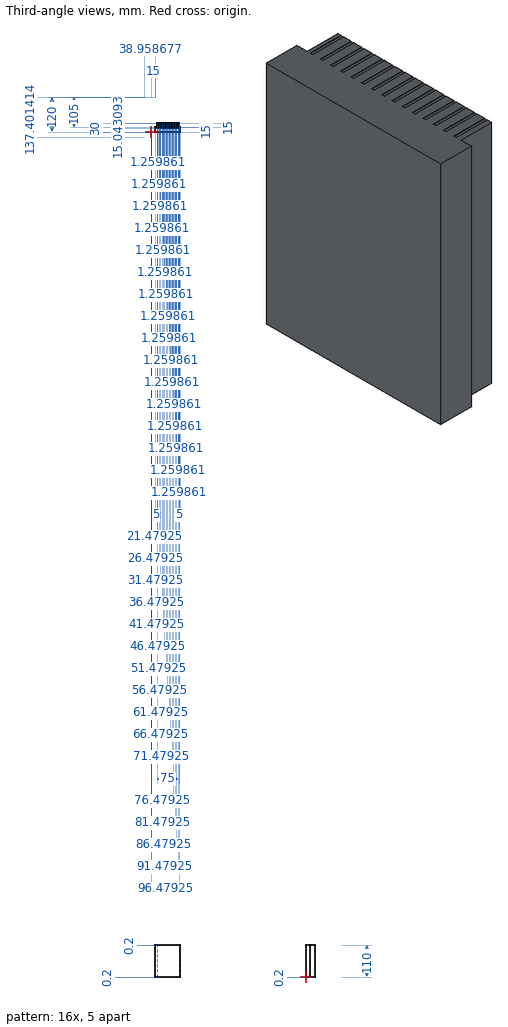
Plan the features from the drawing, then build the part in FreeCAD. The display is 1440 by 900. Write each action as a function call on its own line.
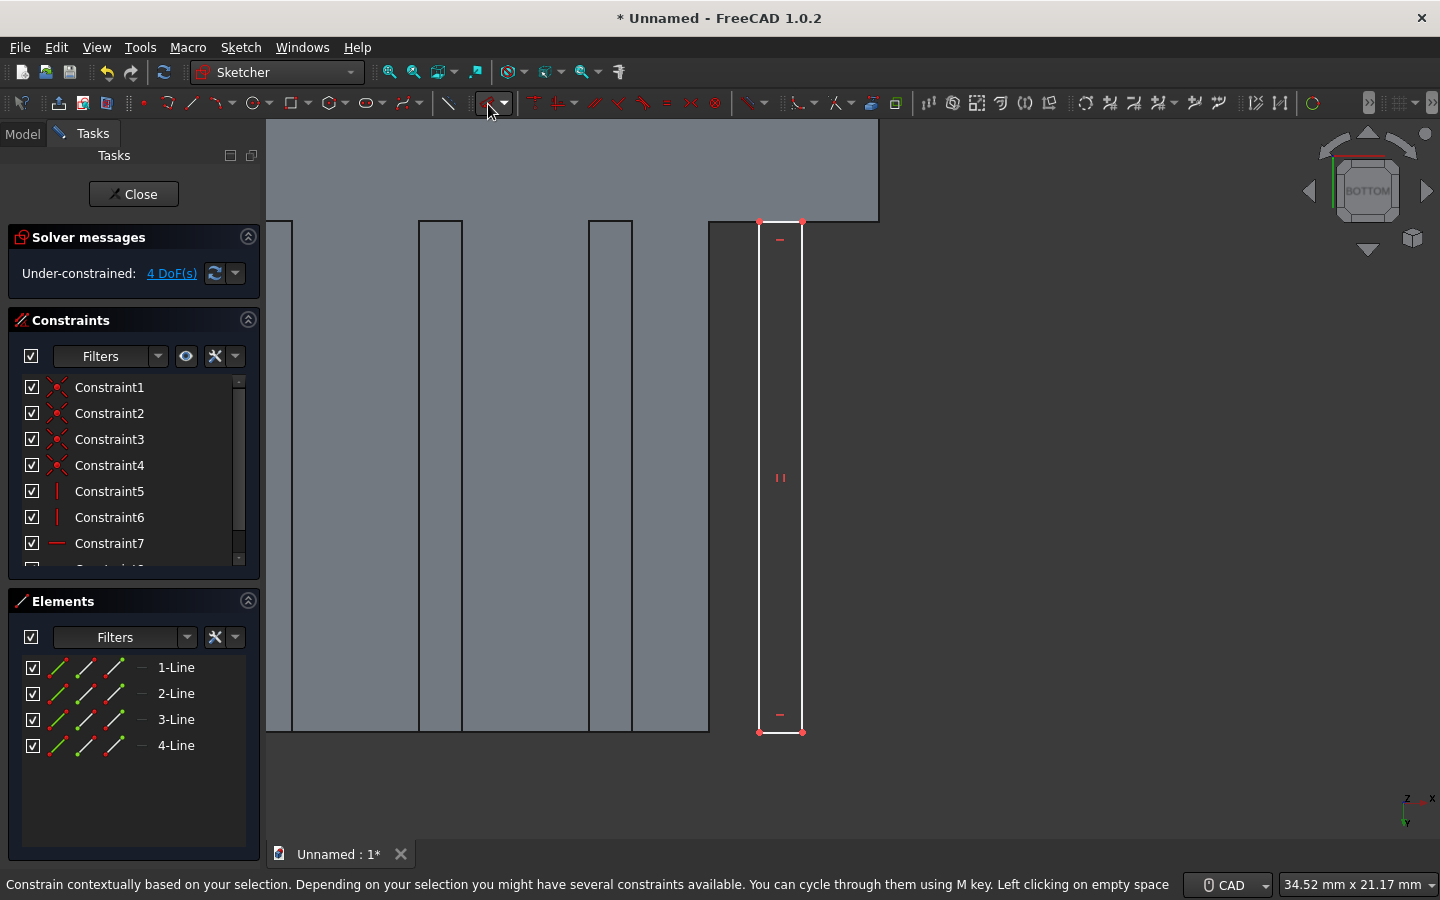
click(759, 733)
click(817, 440)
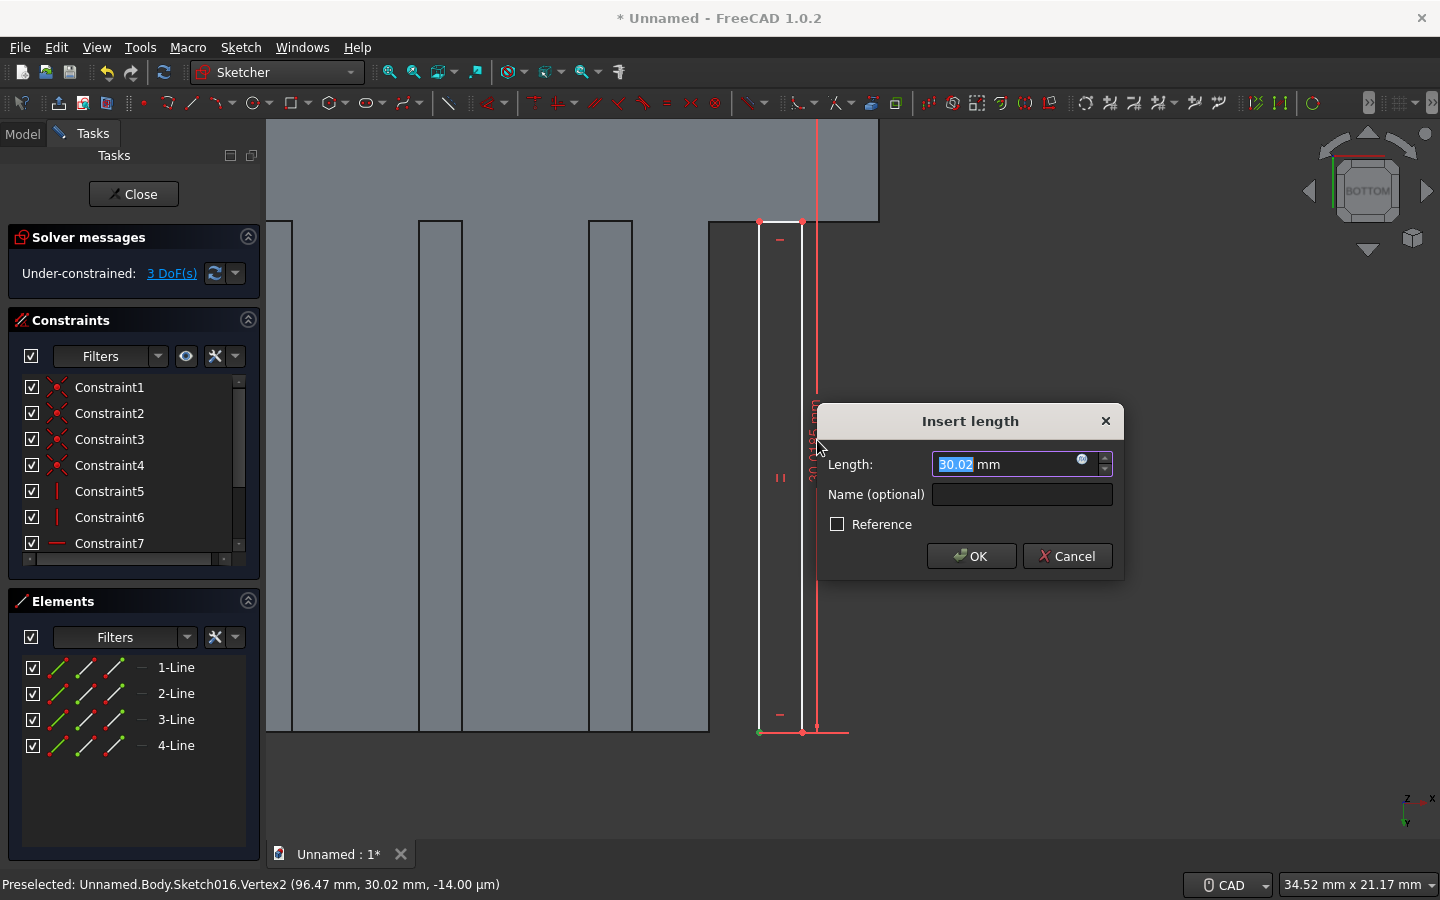
text(30)
key(Return)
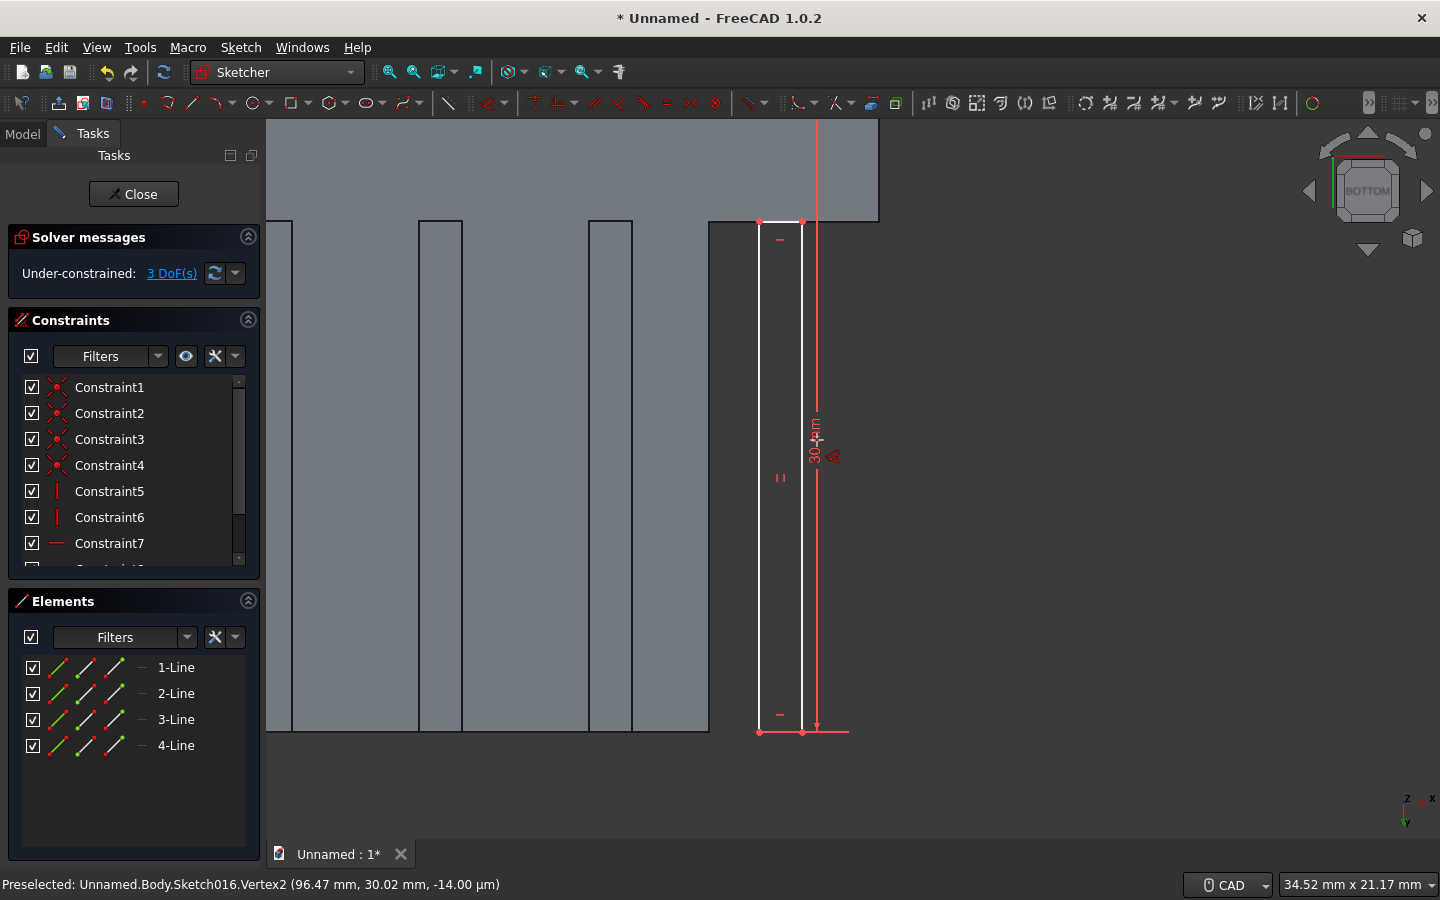
click(772, 732)
click(781, 766)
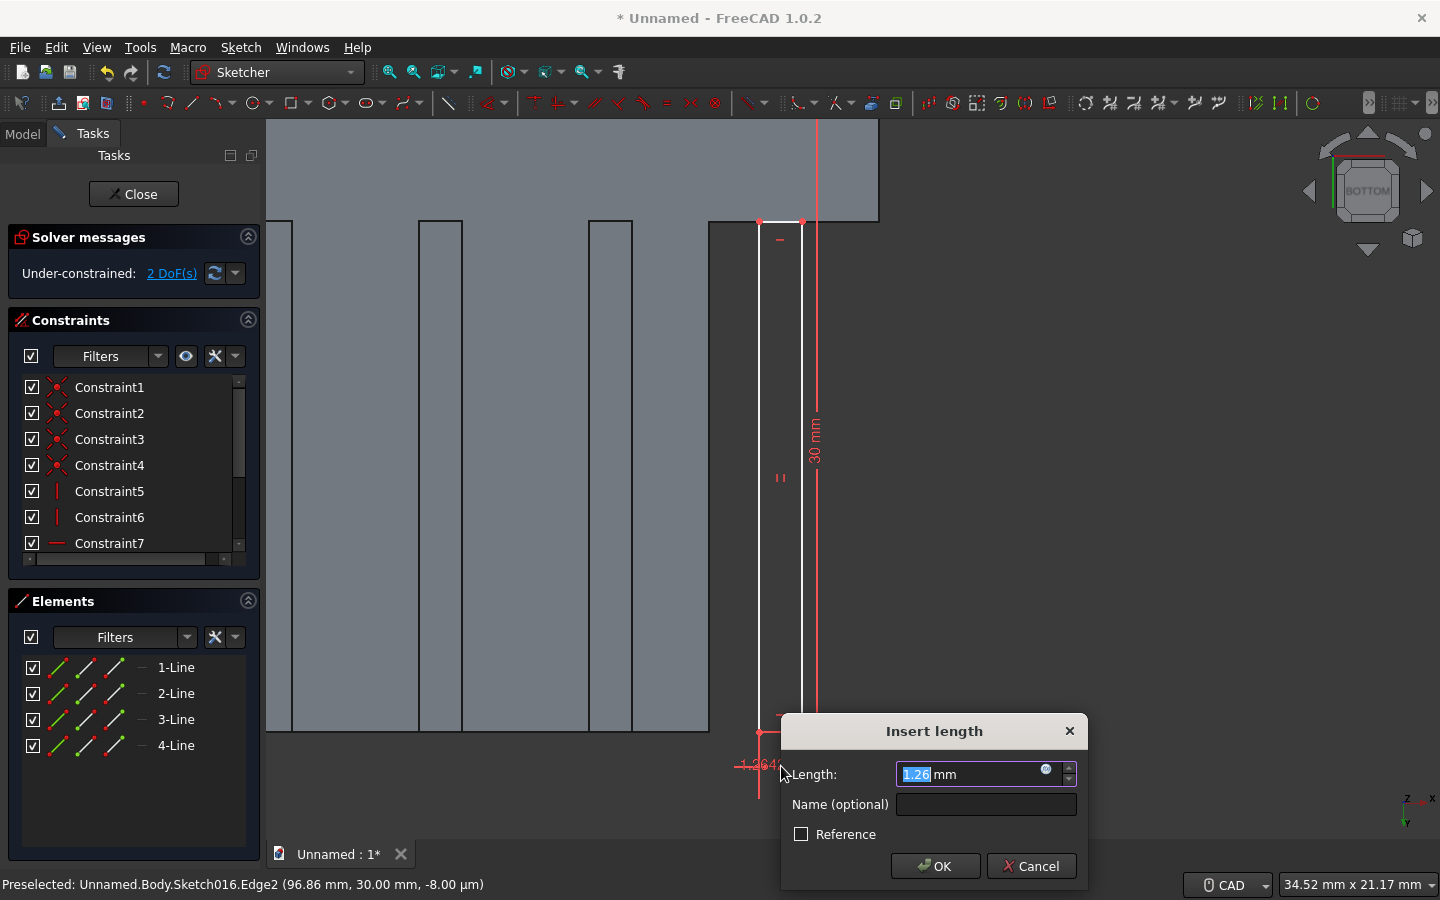
text(1.259861)
key(Return)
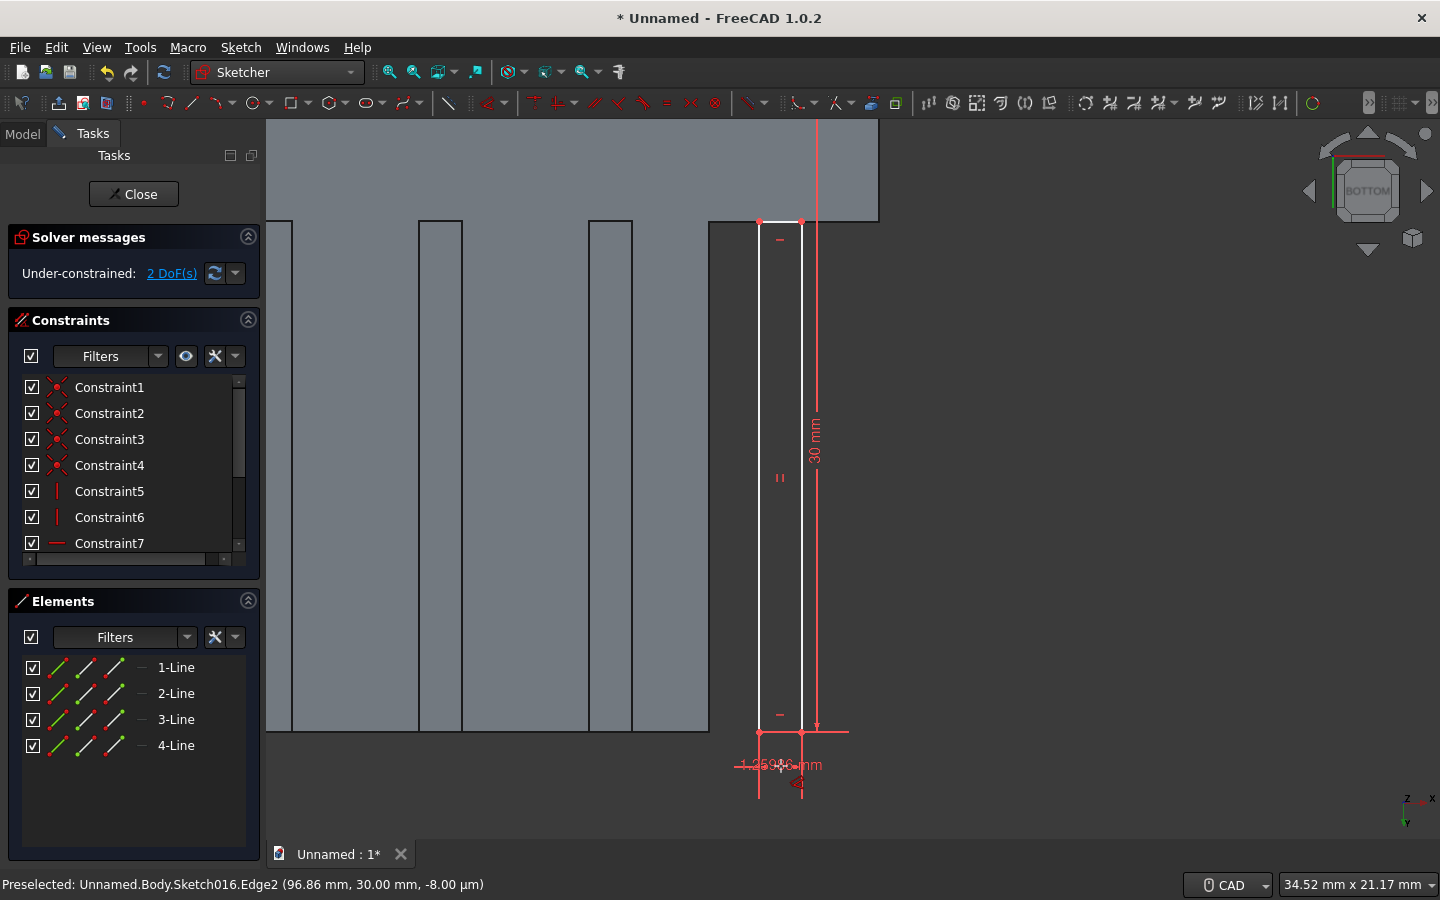
click(759, 375)
click(725, 477)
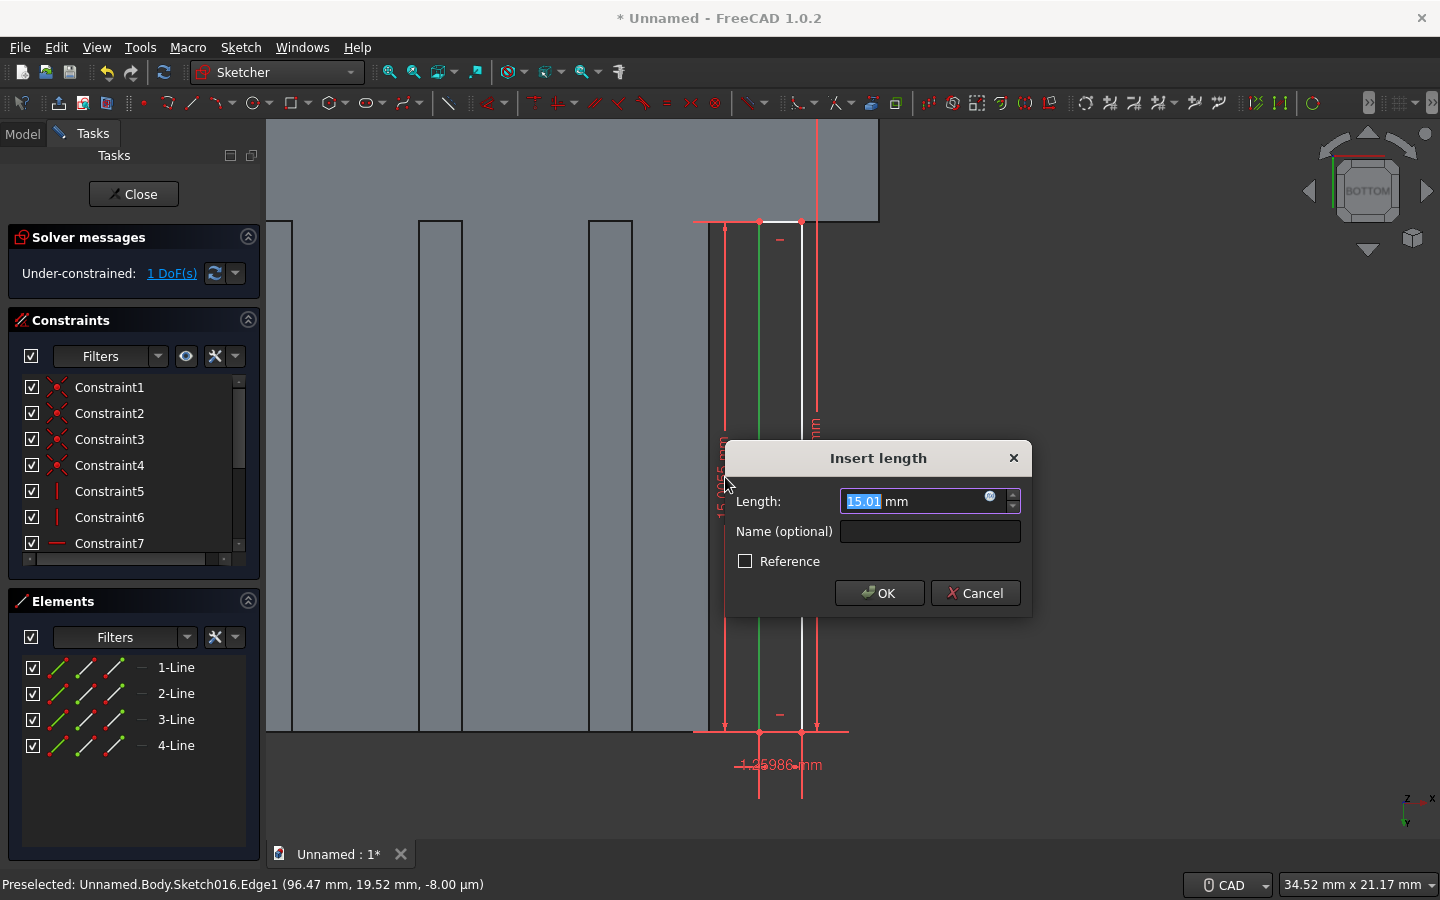
text(15.043093)
key(Return)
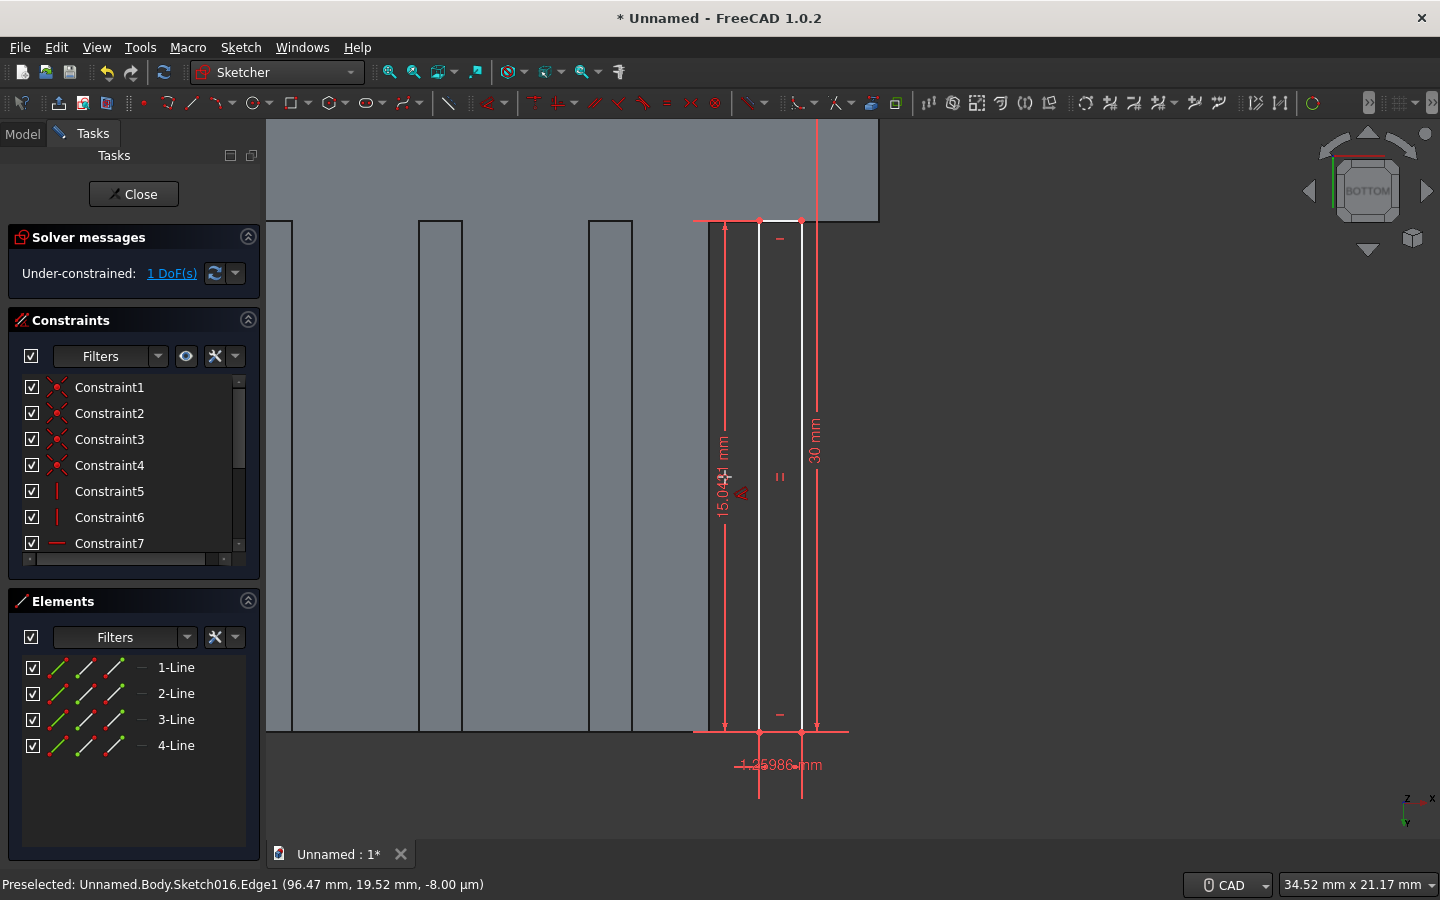
click(759, 221)
click(527, 255)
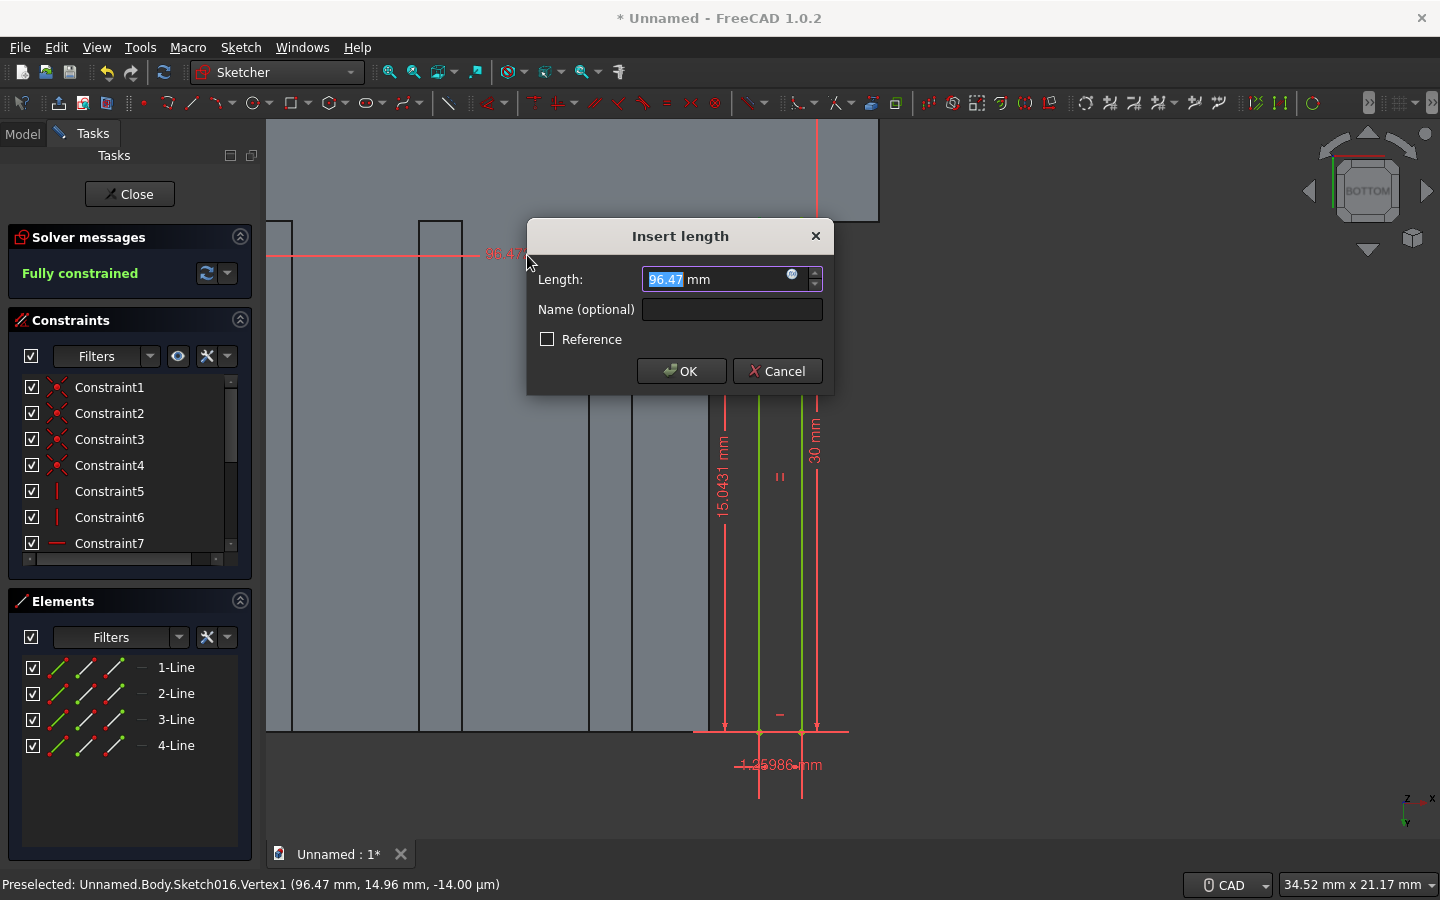
text(96.47925)
key(Return)
key(Escape)